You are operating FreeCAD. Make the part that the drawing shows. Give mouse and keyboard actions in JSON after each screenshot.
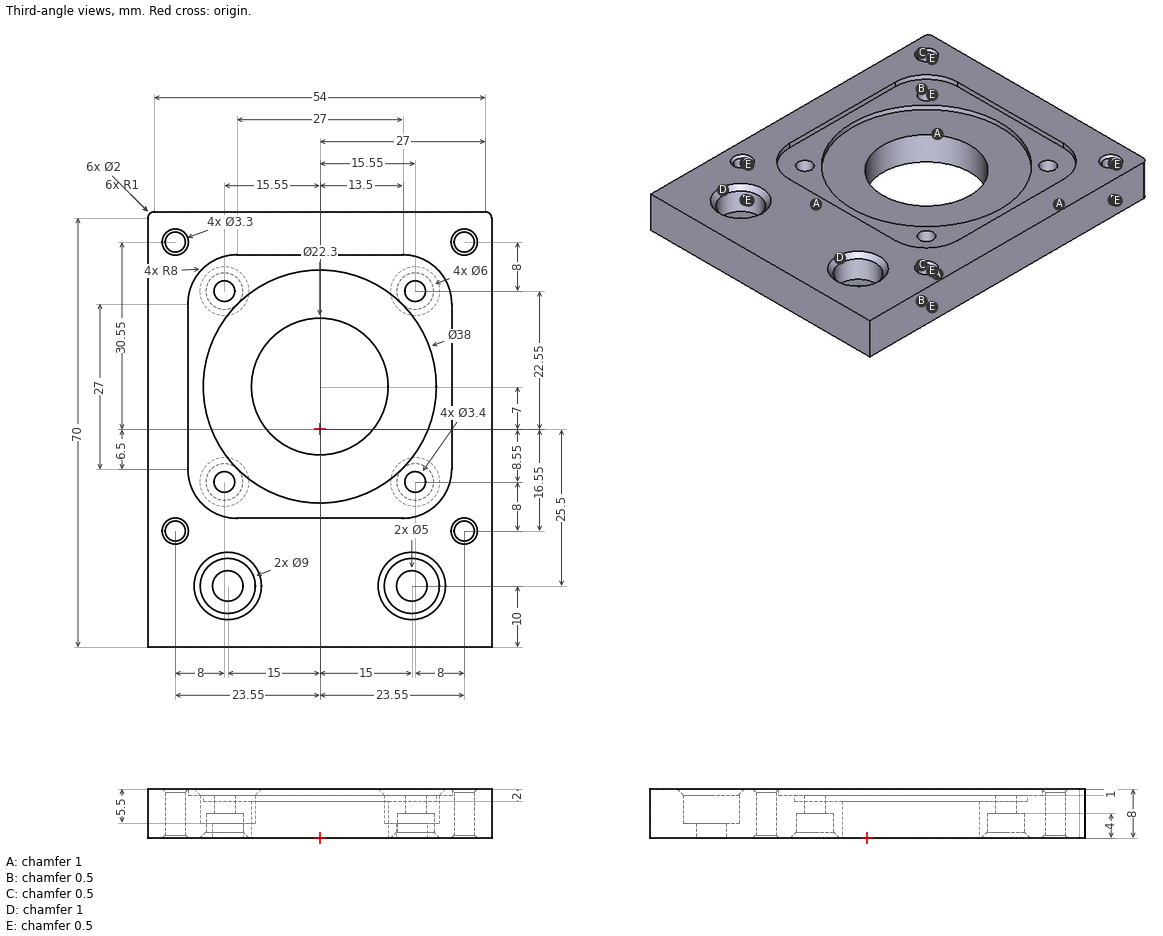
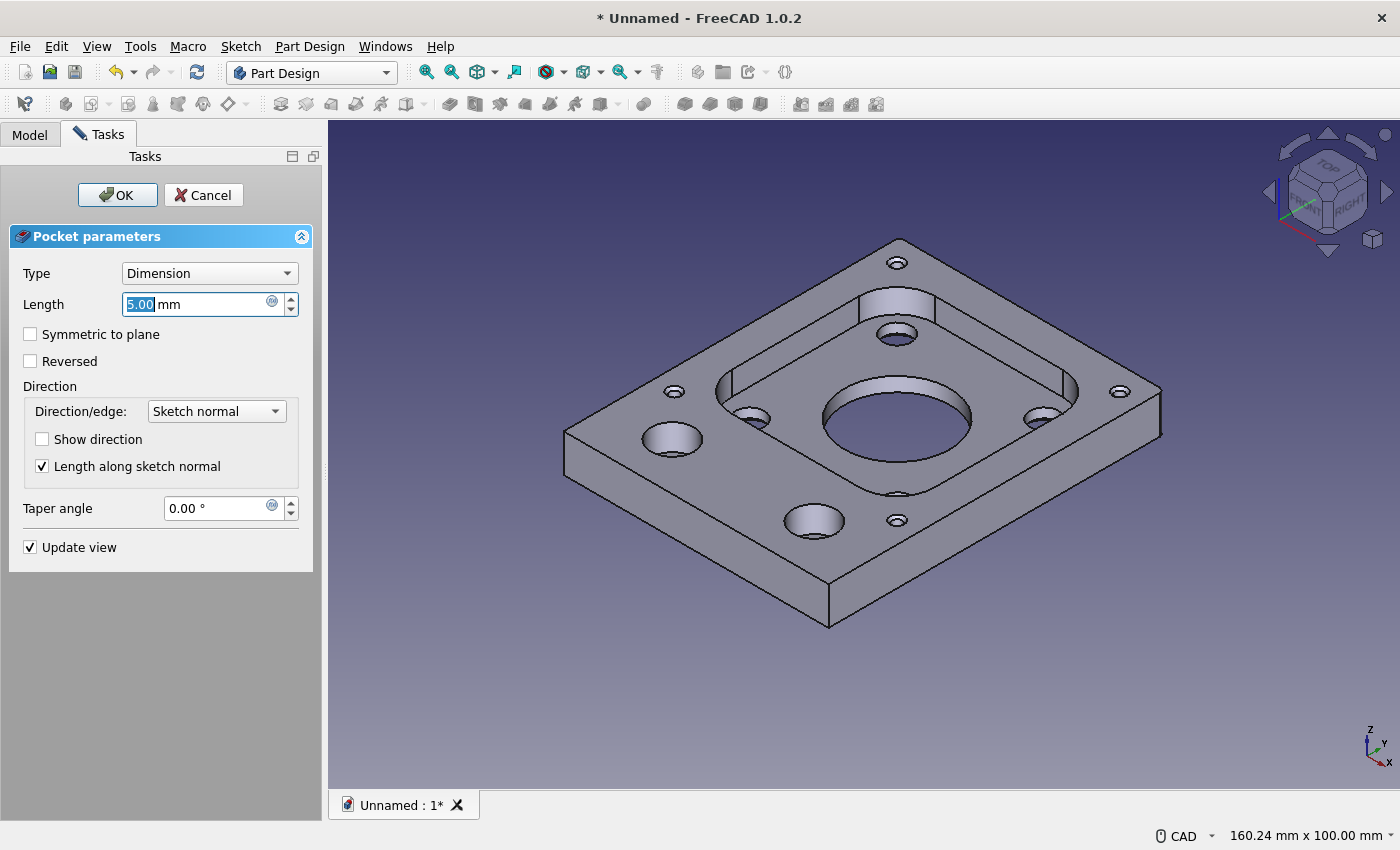
{"action": "type", "text": "1"}
{"action": "key", "text": "Tab"}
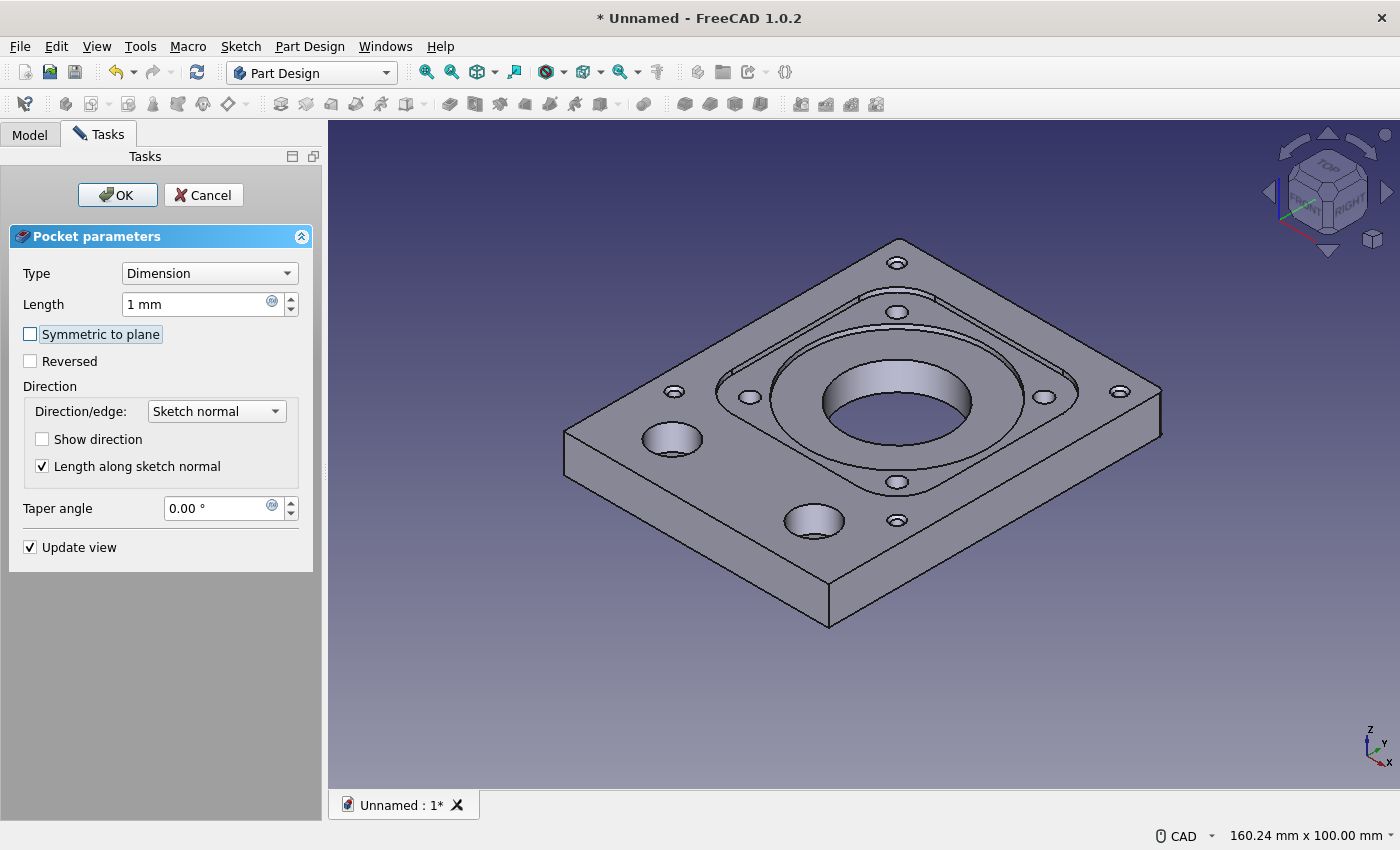
{"action": "left_click", "coordinate": [118, 195]}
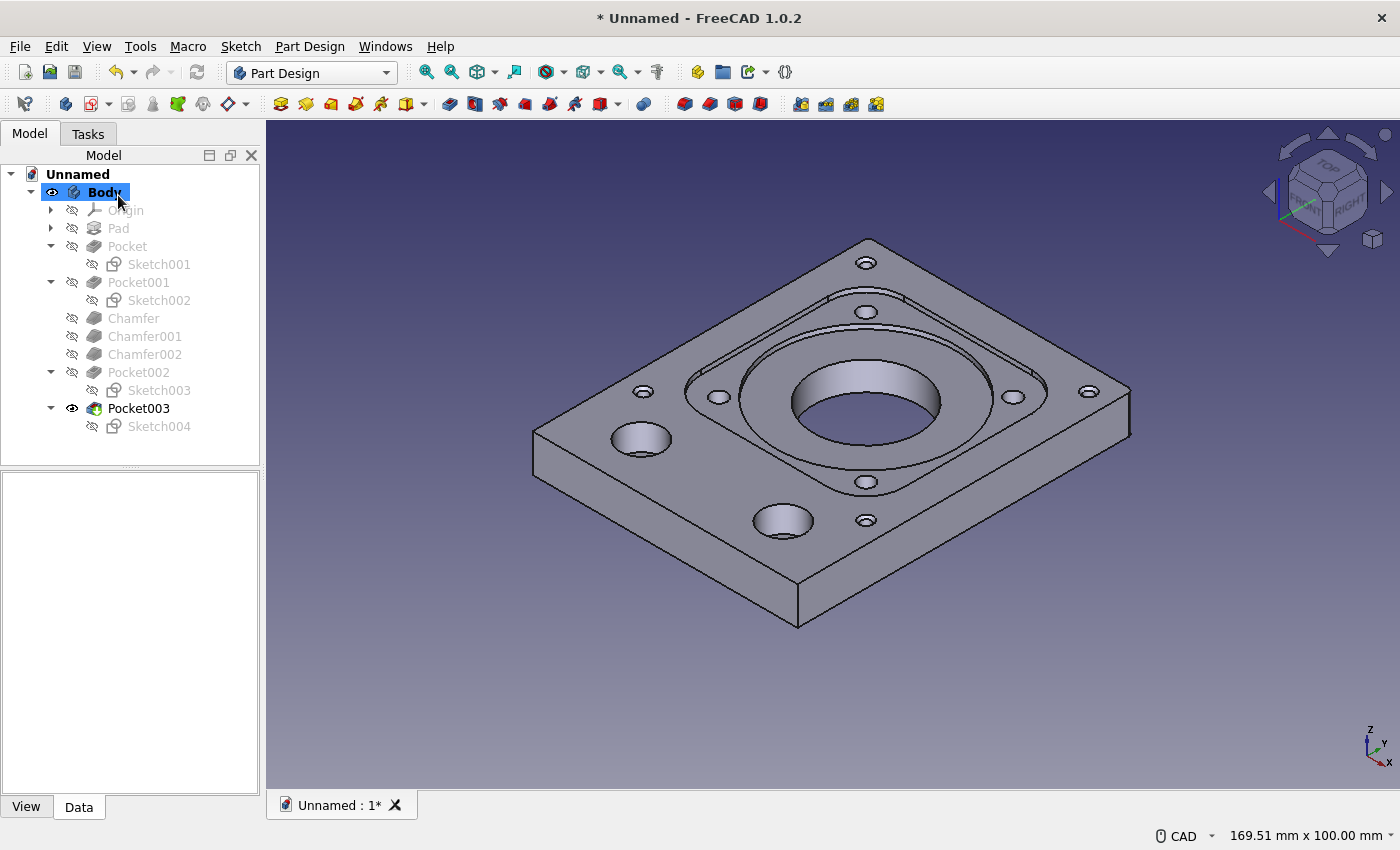
{"action": "left_click", "coordinate": [620, 426]}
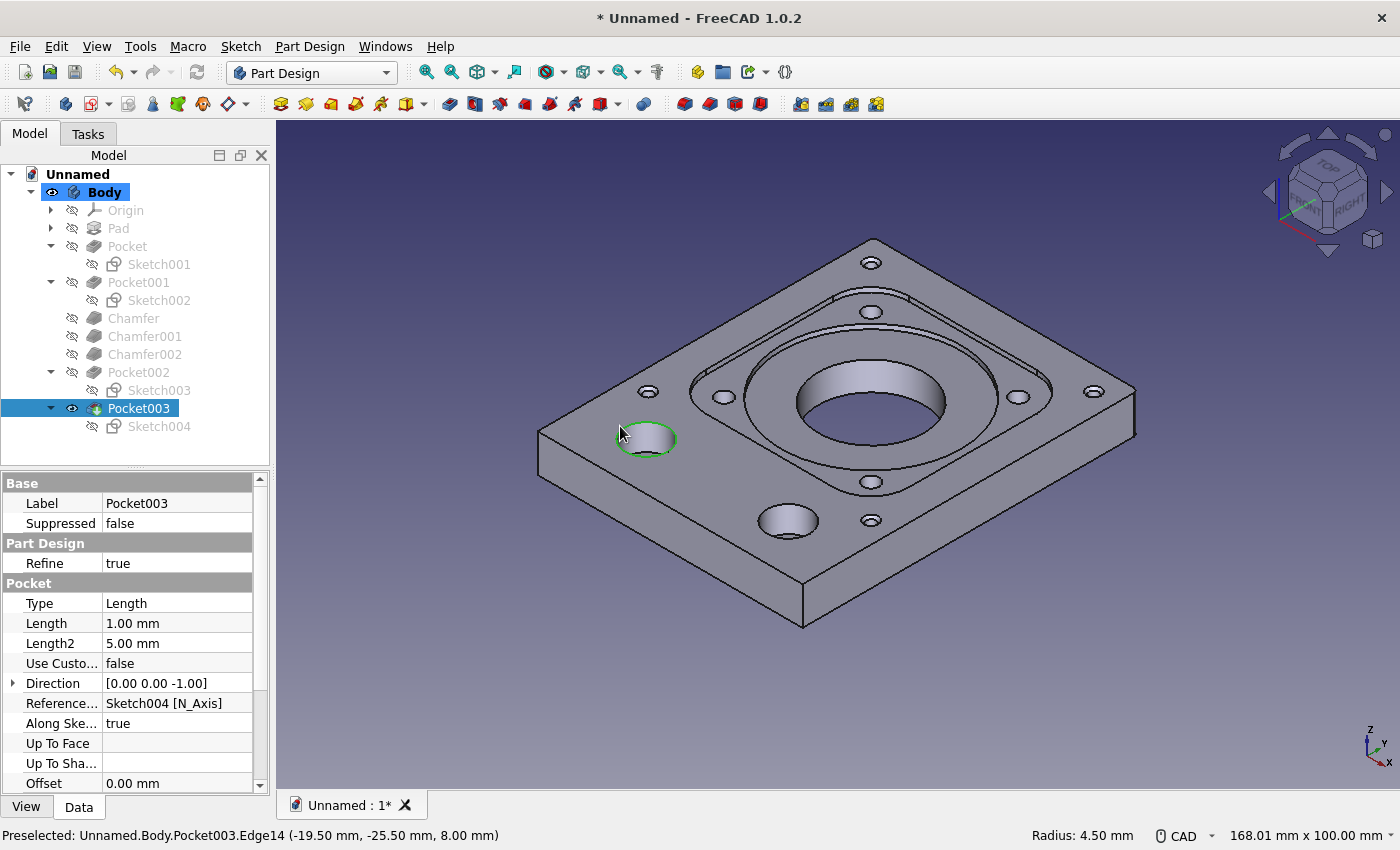
{"action": "left_click", "coordinate": [767, 508], "text": "ctrl"}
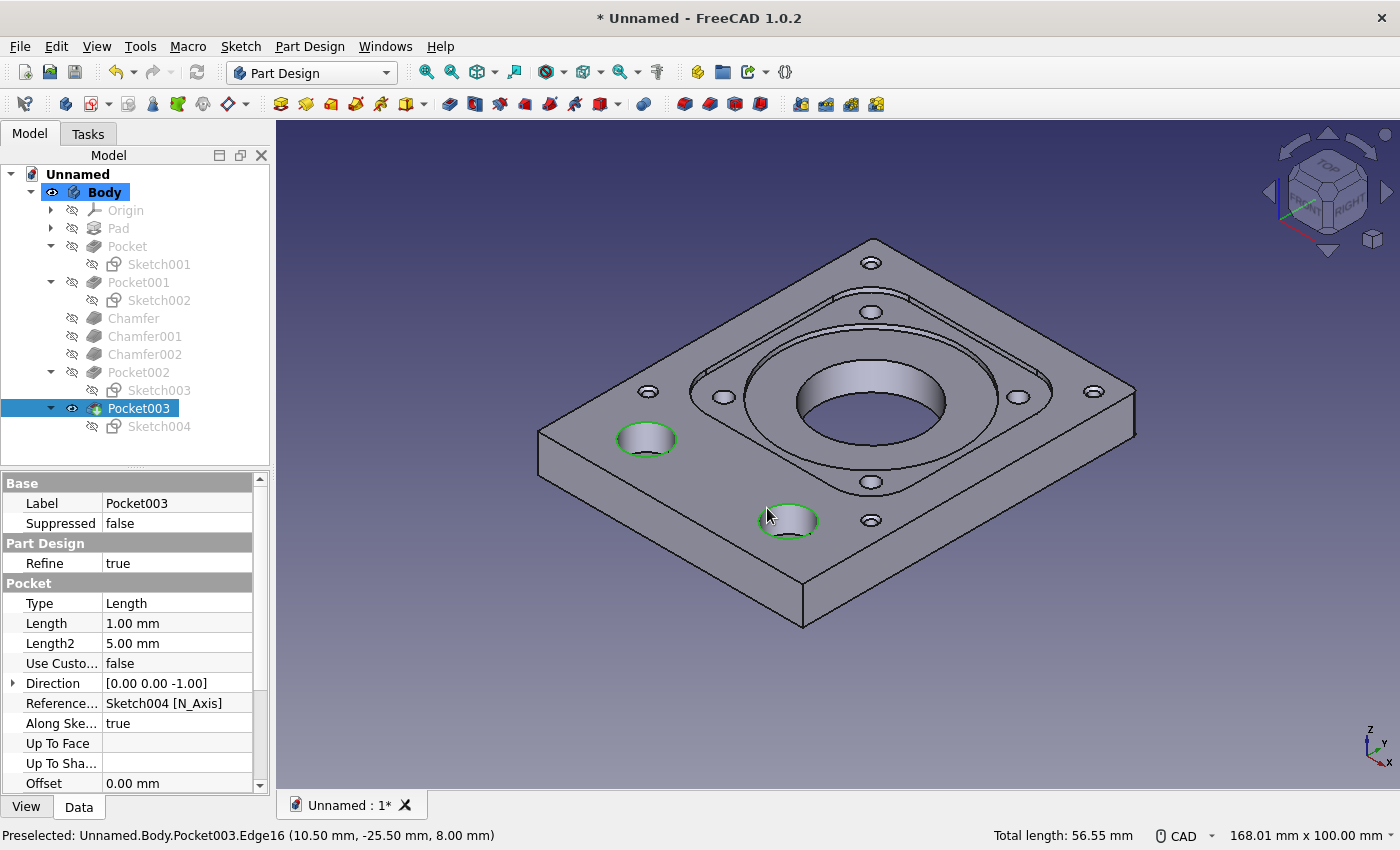
{"action": "left_click", "coordinate": [710, 104]}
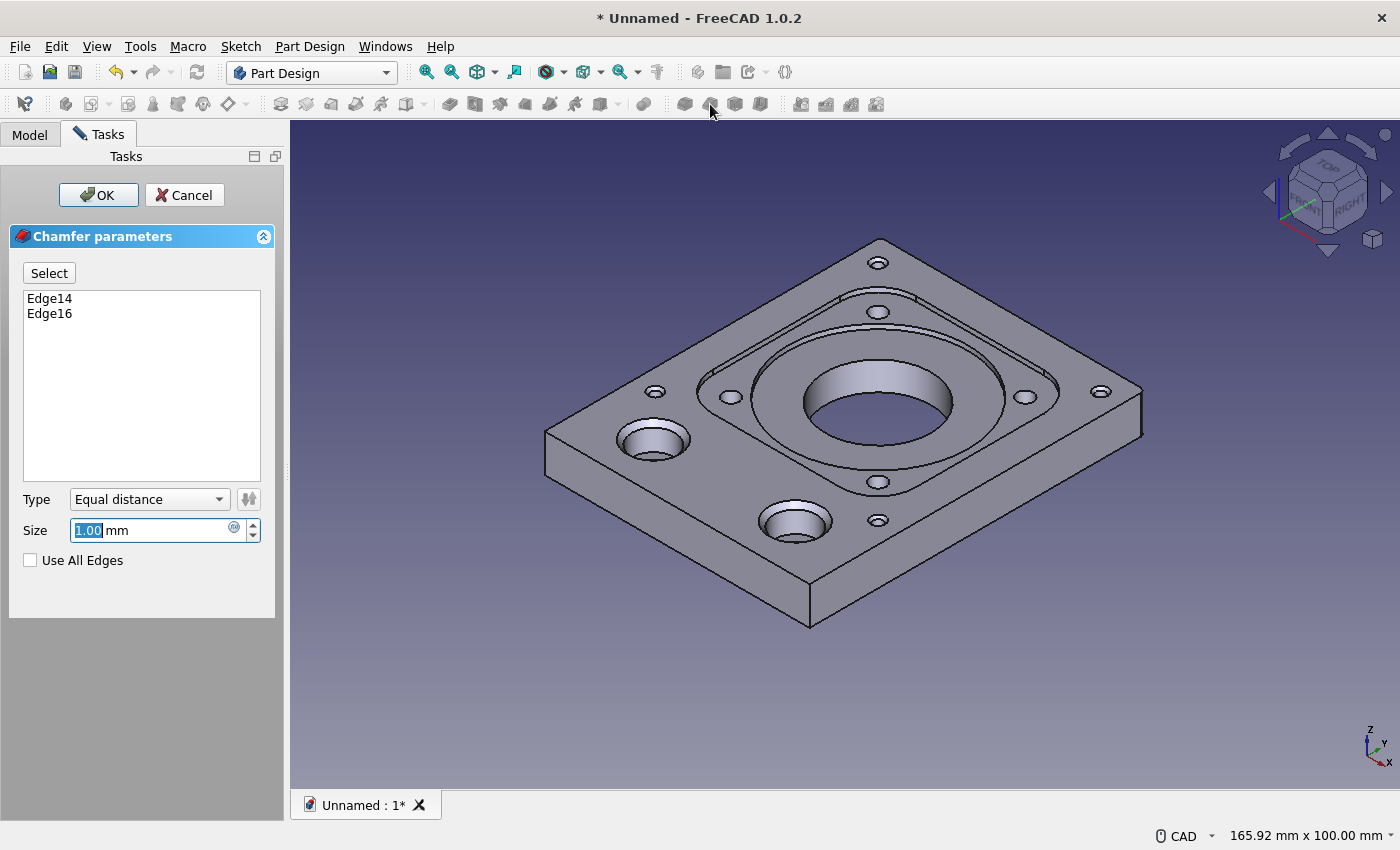
{"action": "type", "text": "1"}
{"action": "key", "text": "Tab"}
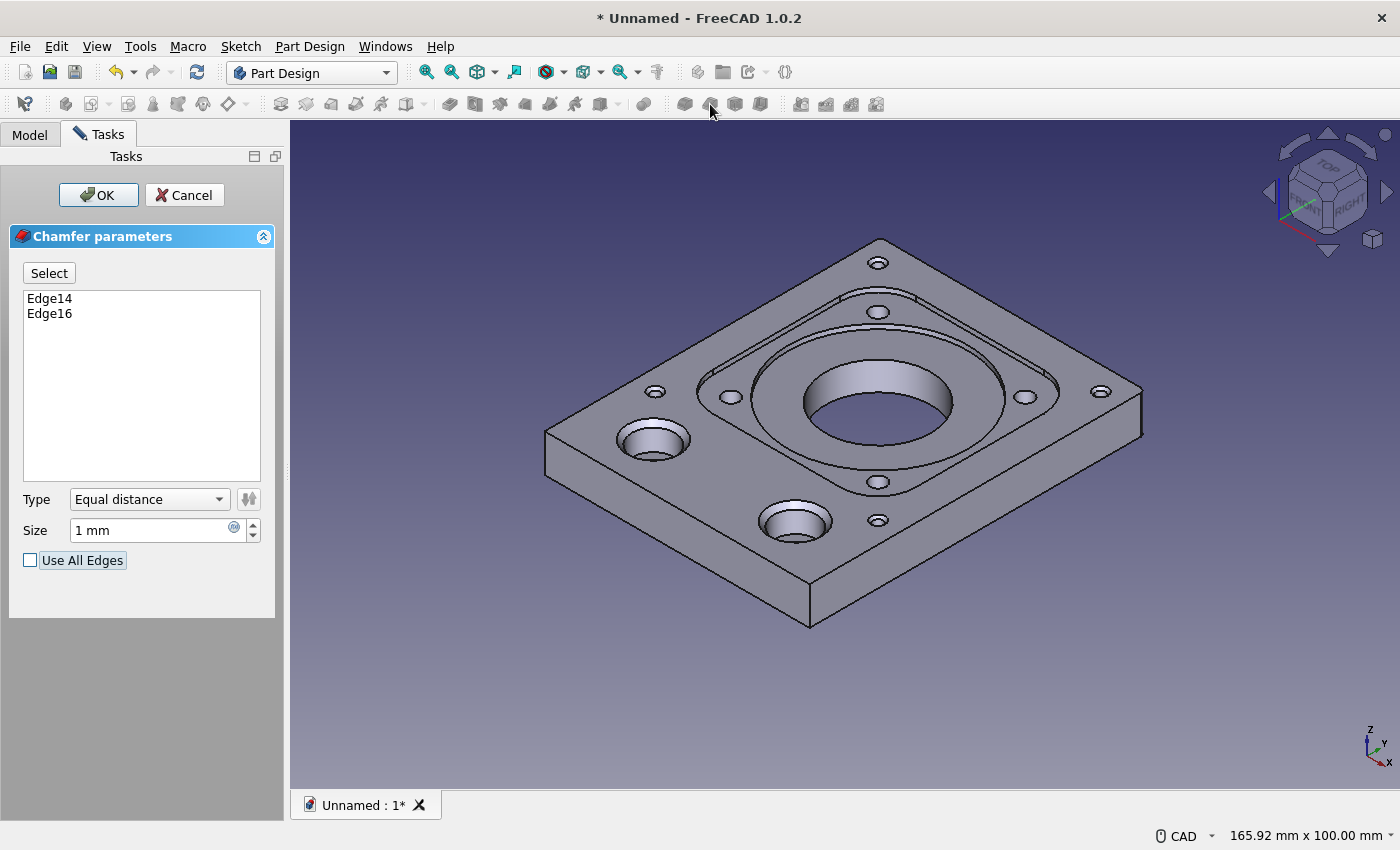
{"action": "left_click", "coordinate": [99, 195]}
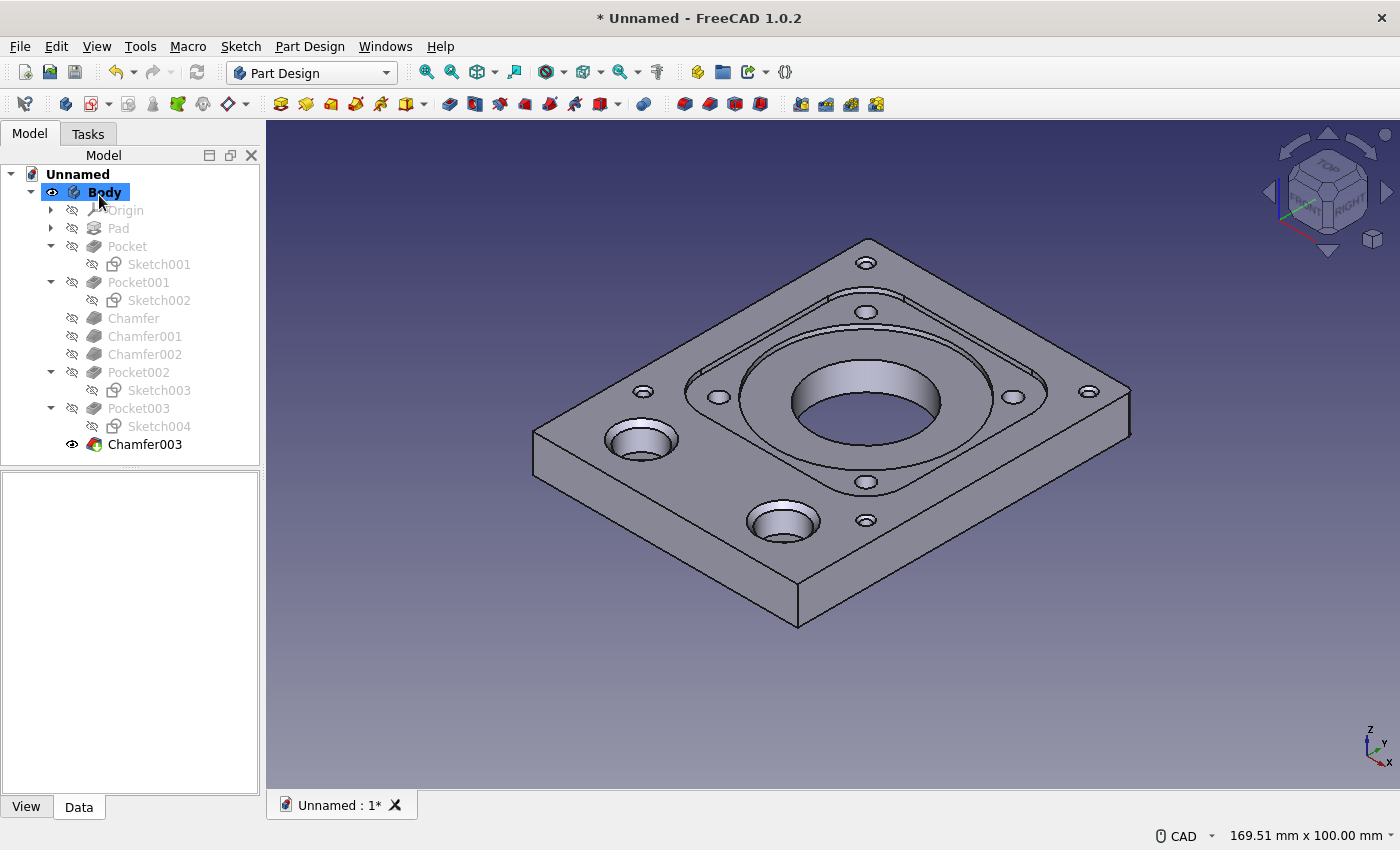
{"action": "left_click", "coordinate": [737, 465]}